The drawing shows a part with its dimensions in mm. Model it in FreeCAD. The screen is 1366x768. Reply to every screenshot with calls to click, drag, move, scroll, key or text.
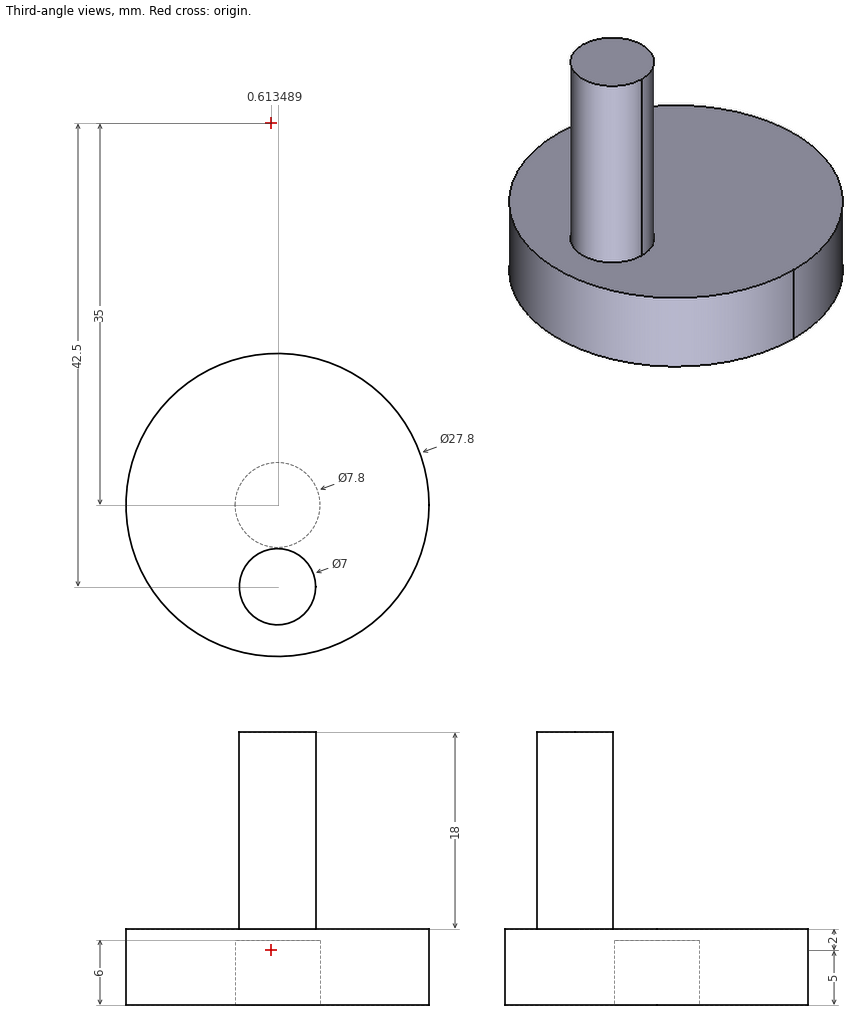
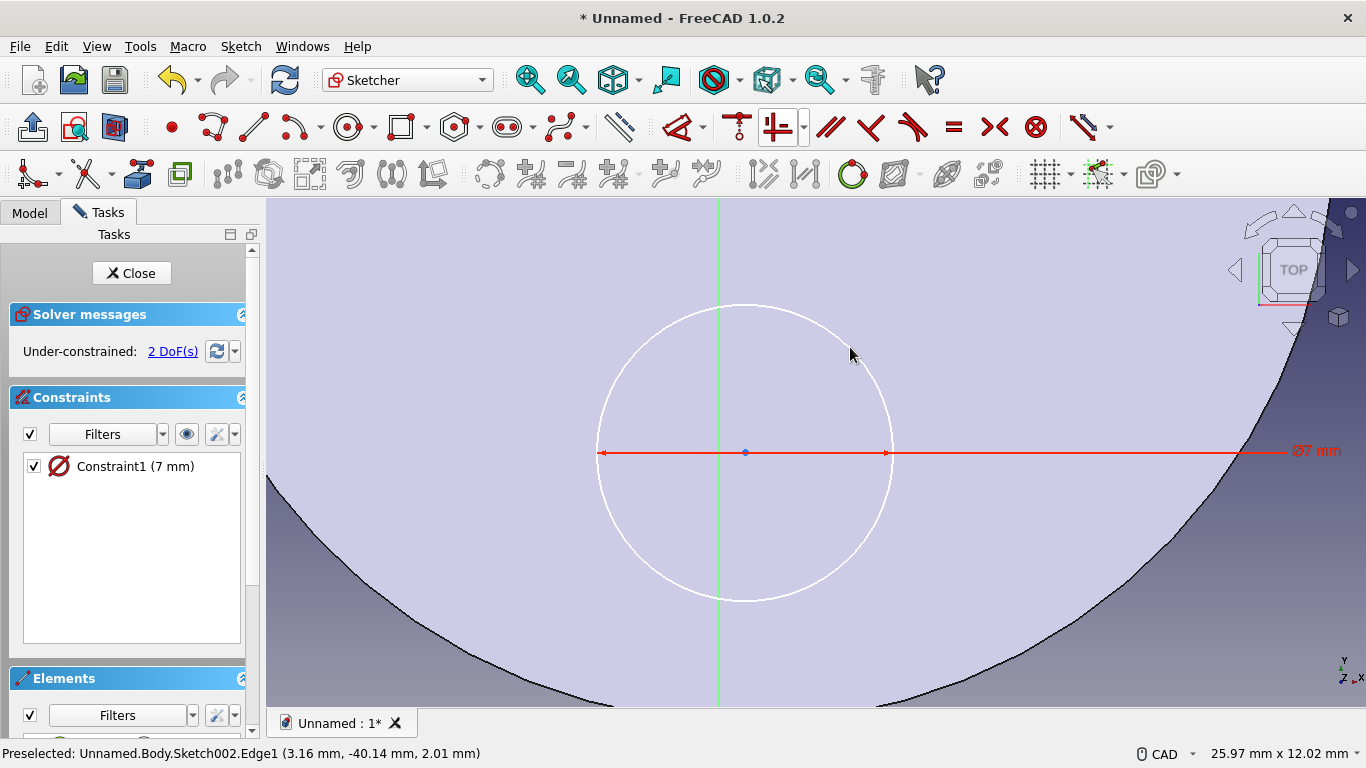
click(676, 128)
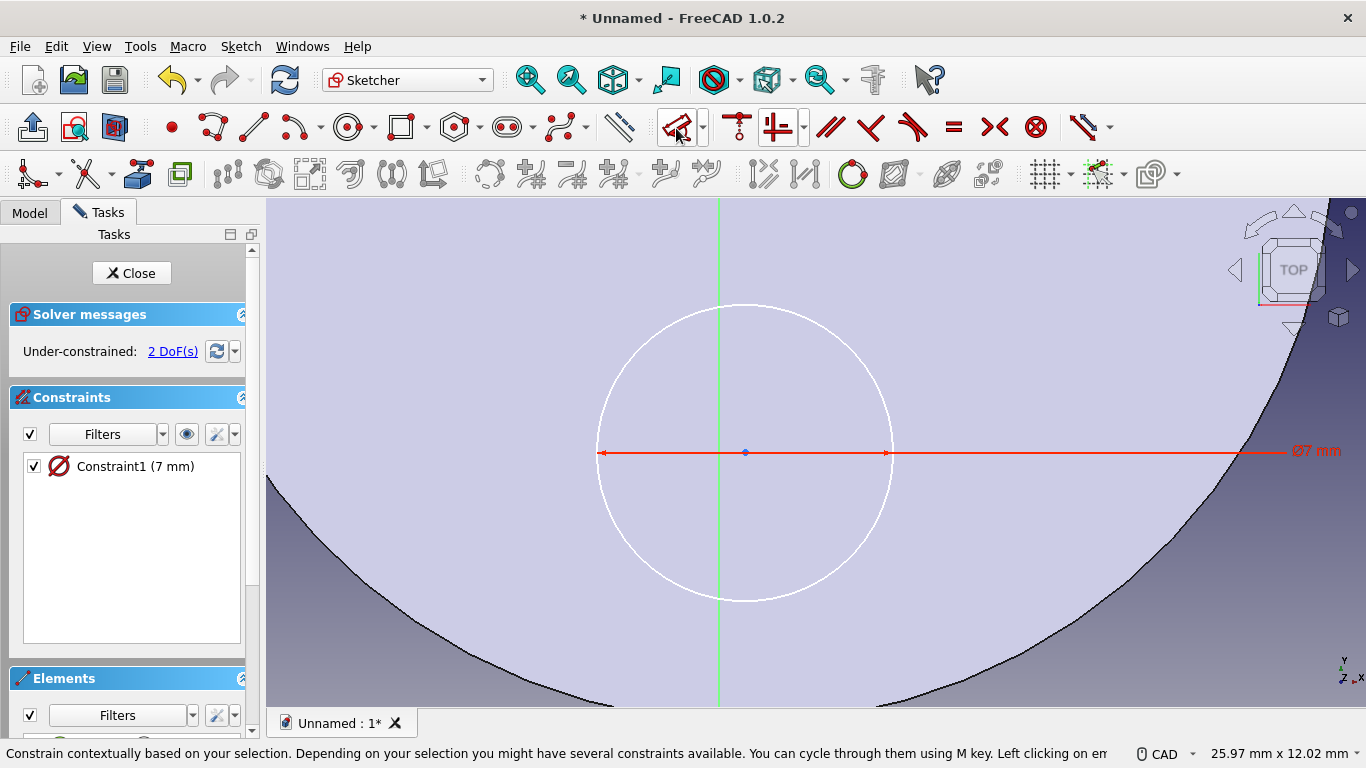
click(745, 453)
click(685, 339)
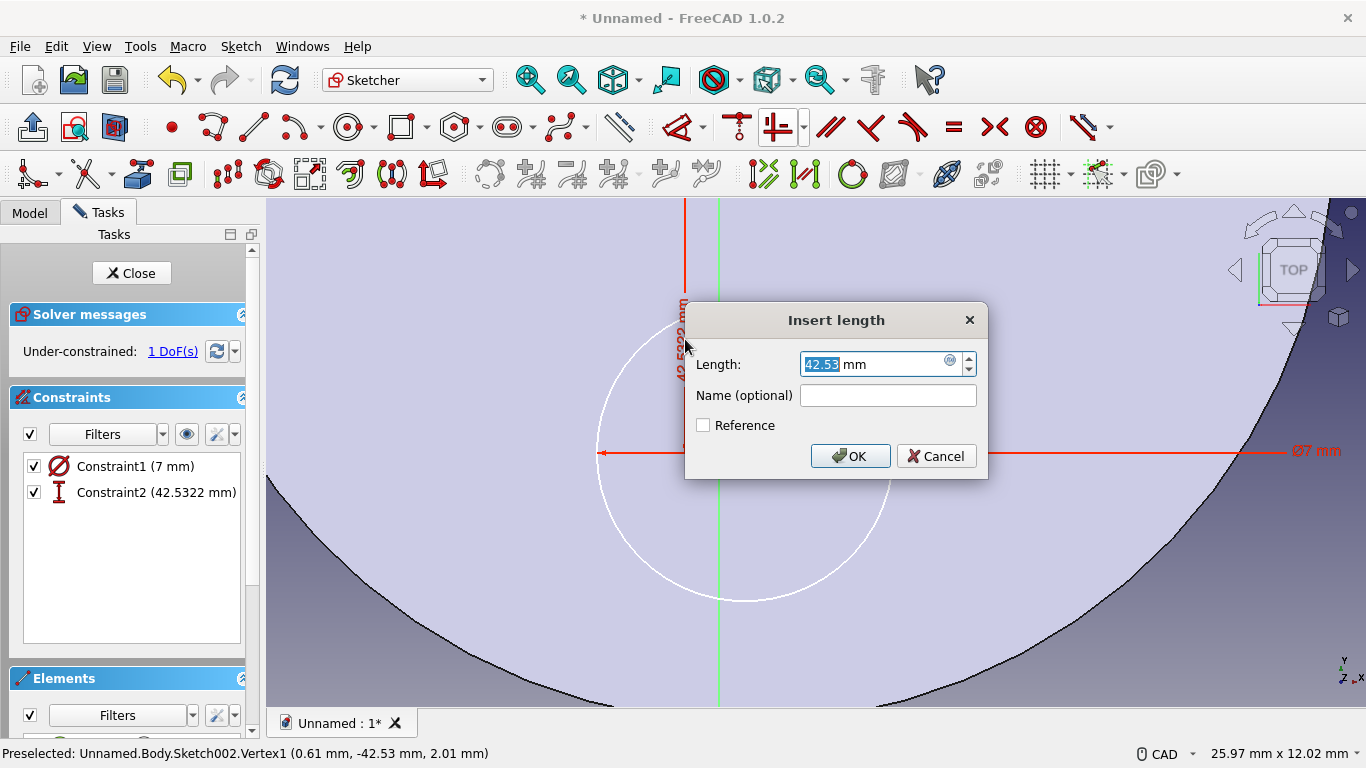
text(42.5)
key(Return)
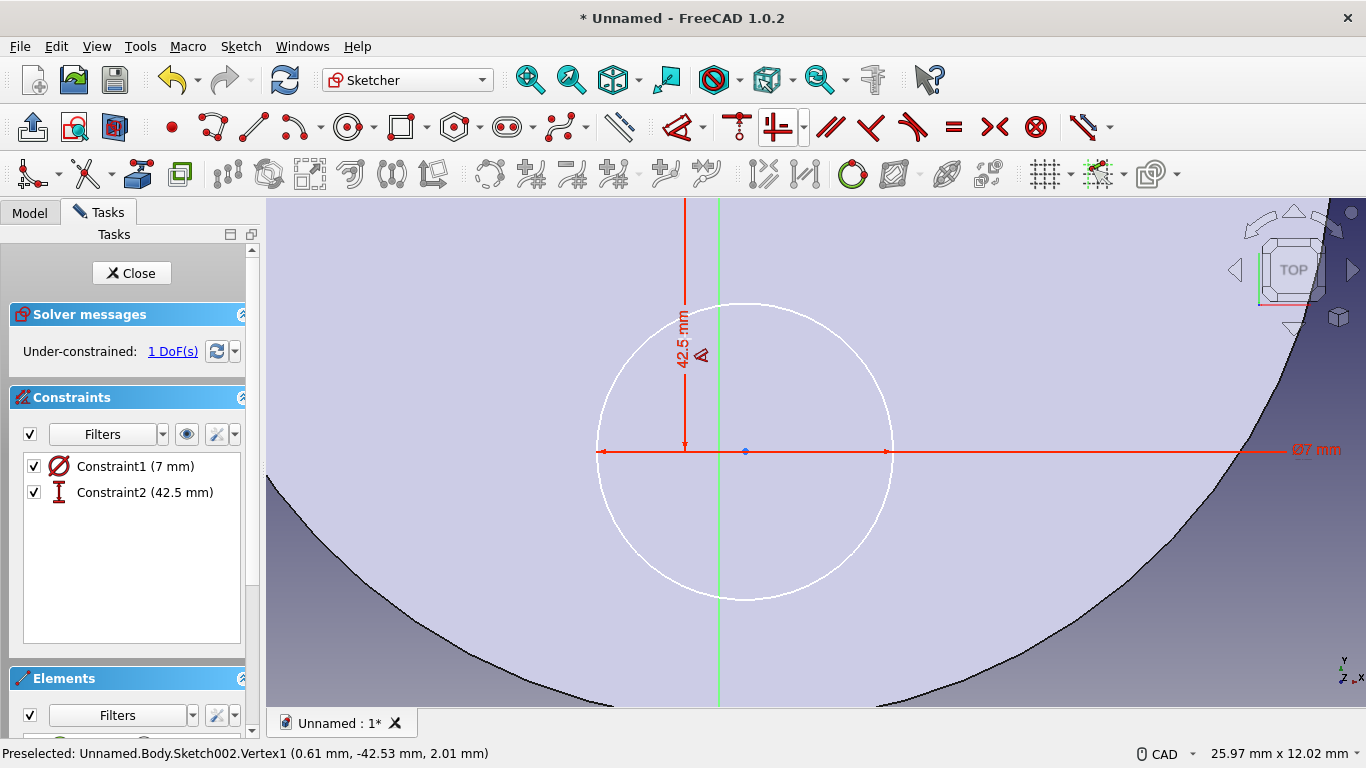
scroll(745, 452, up, 3)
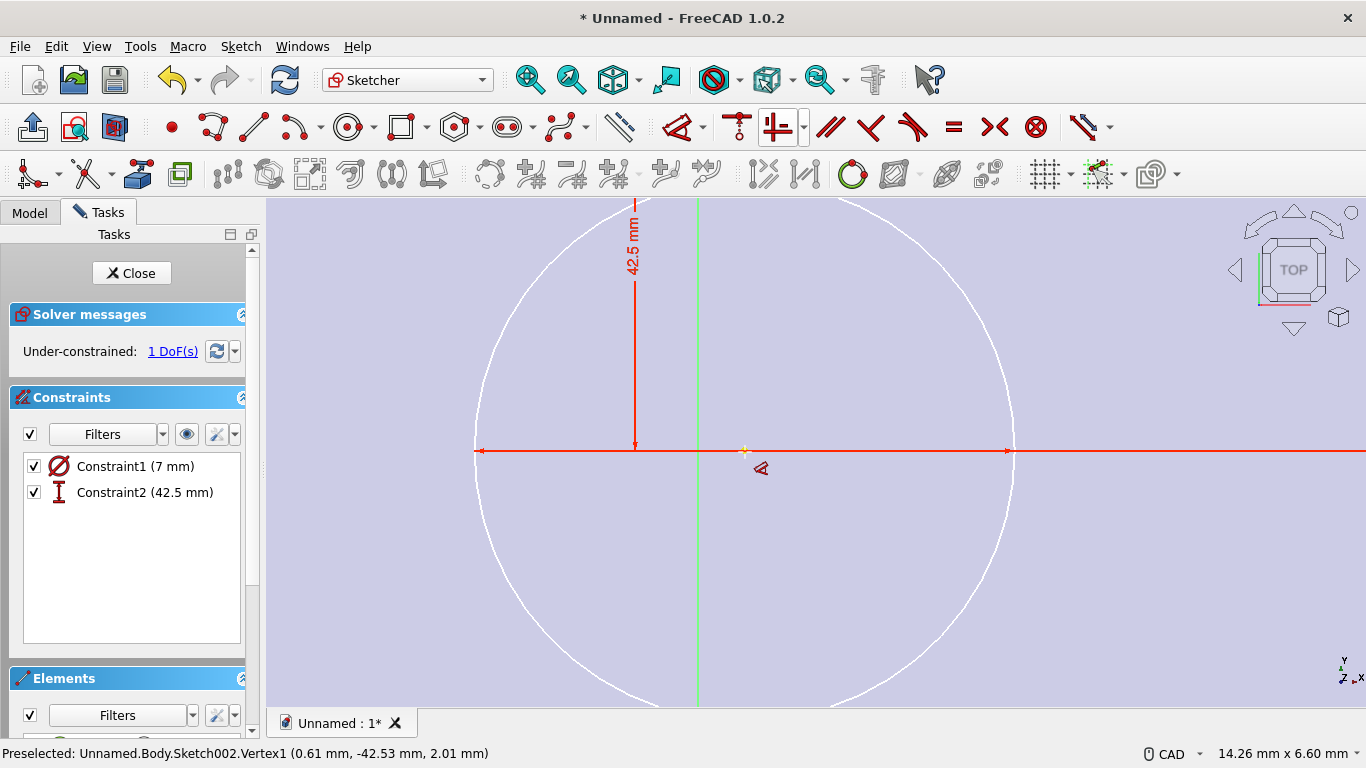
click(745, 451)
click(721, 485)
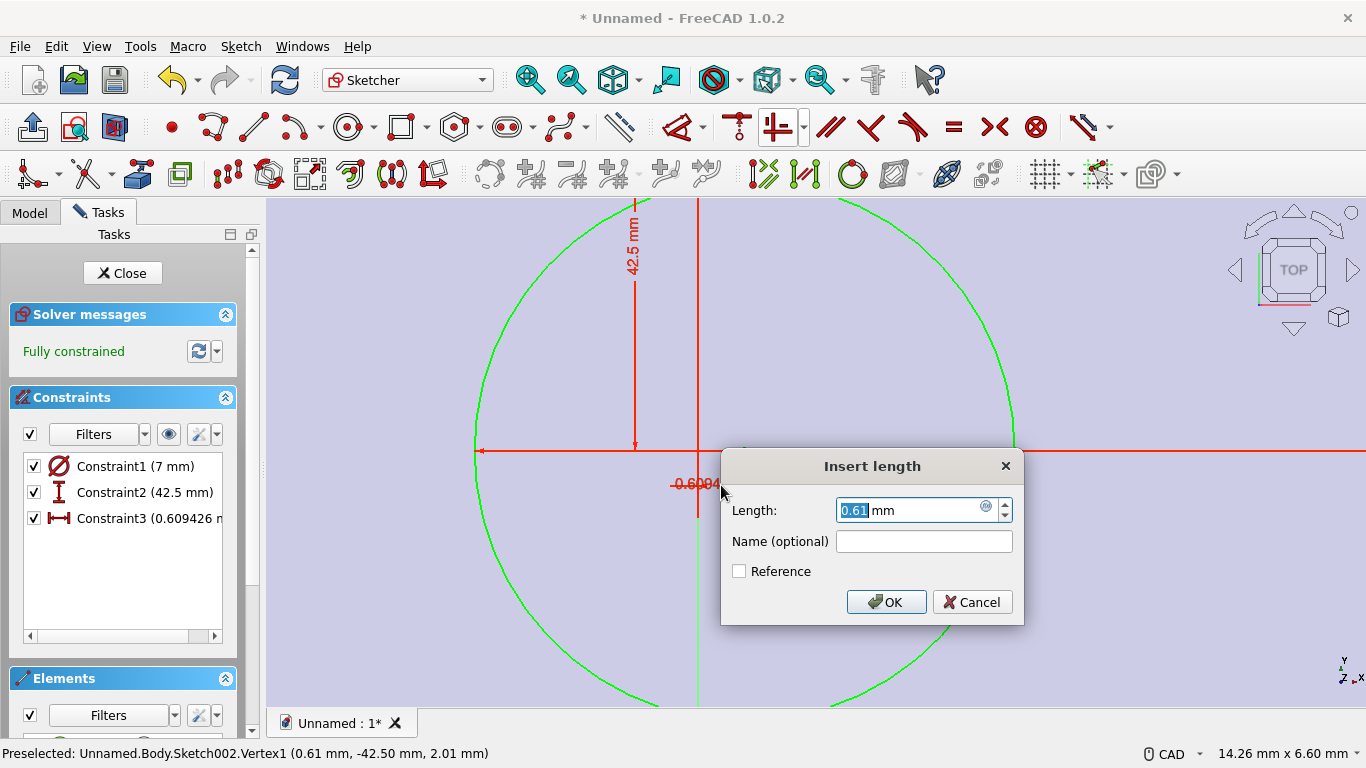
text(0.613489)
key(Return)
key(Escape)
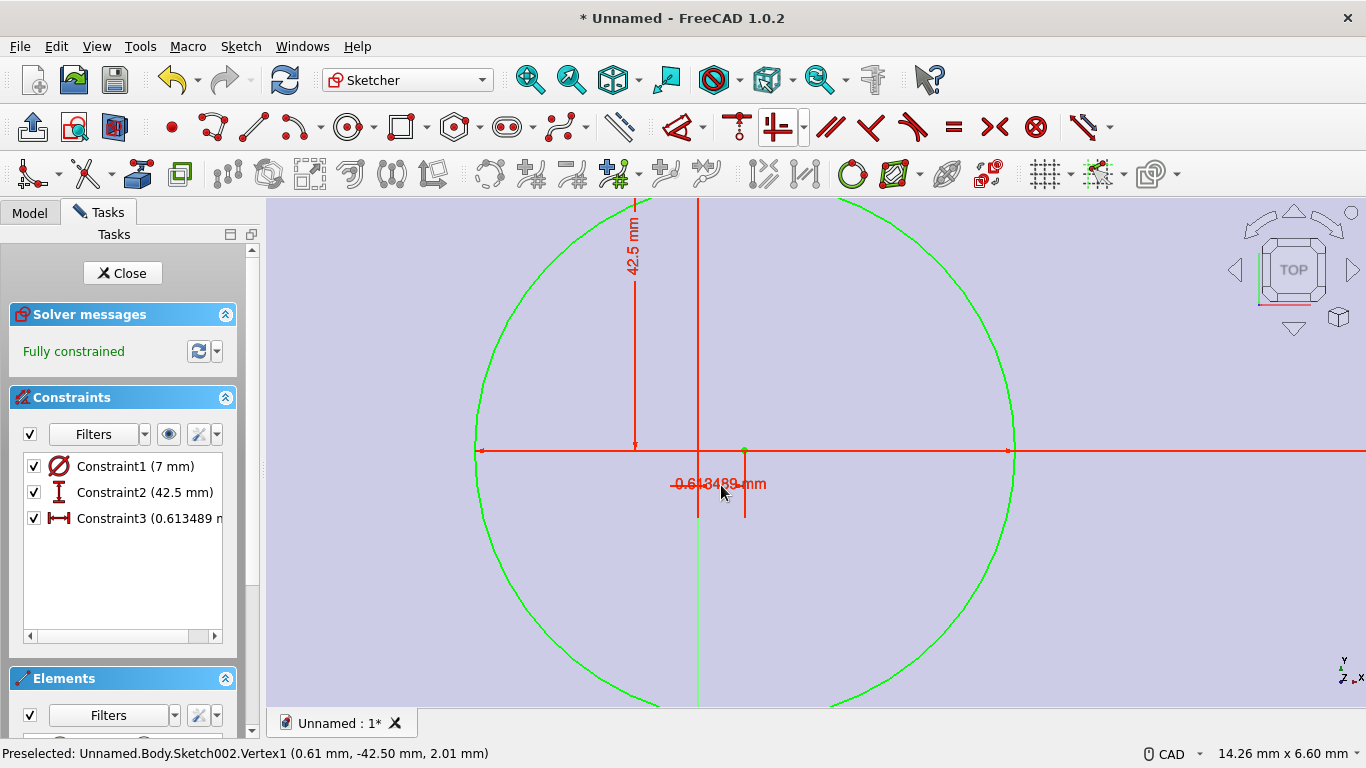
click(123, 273)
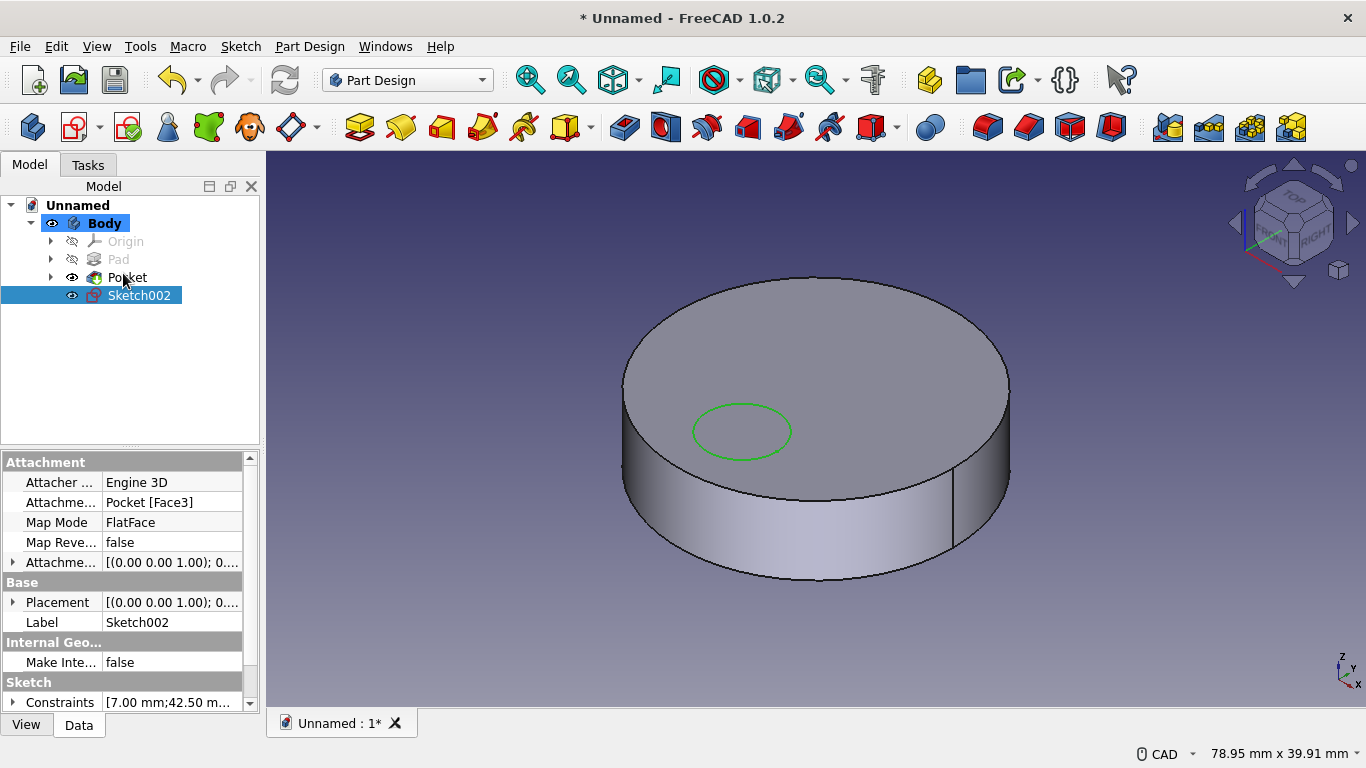
click(360, 128)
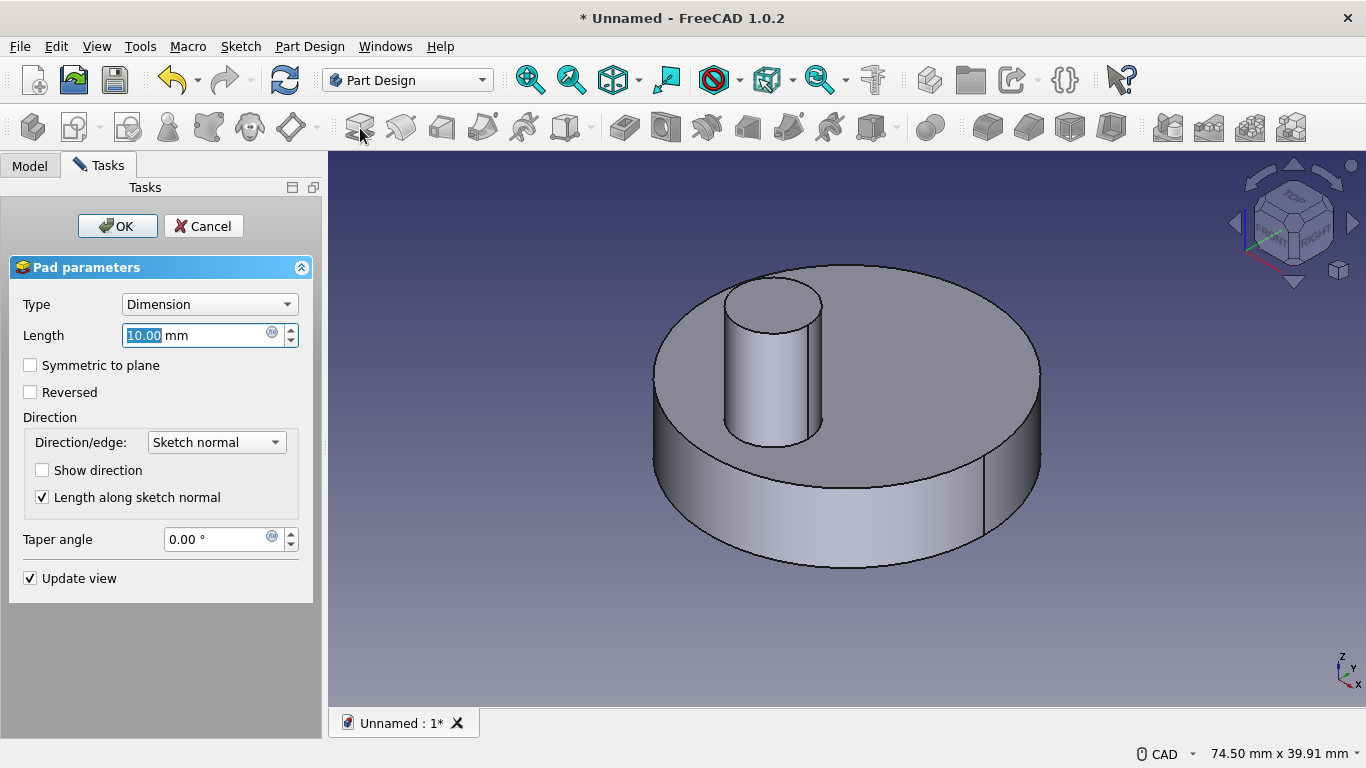
text(18)
key(Tab)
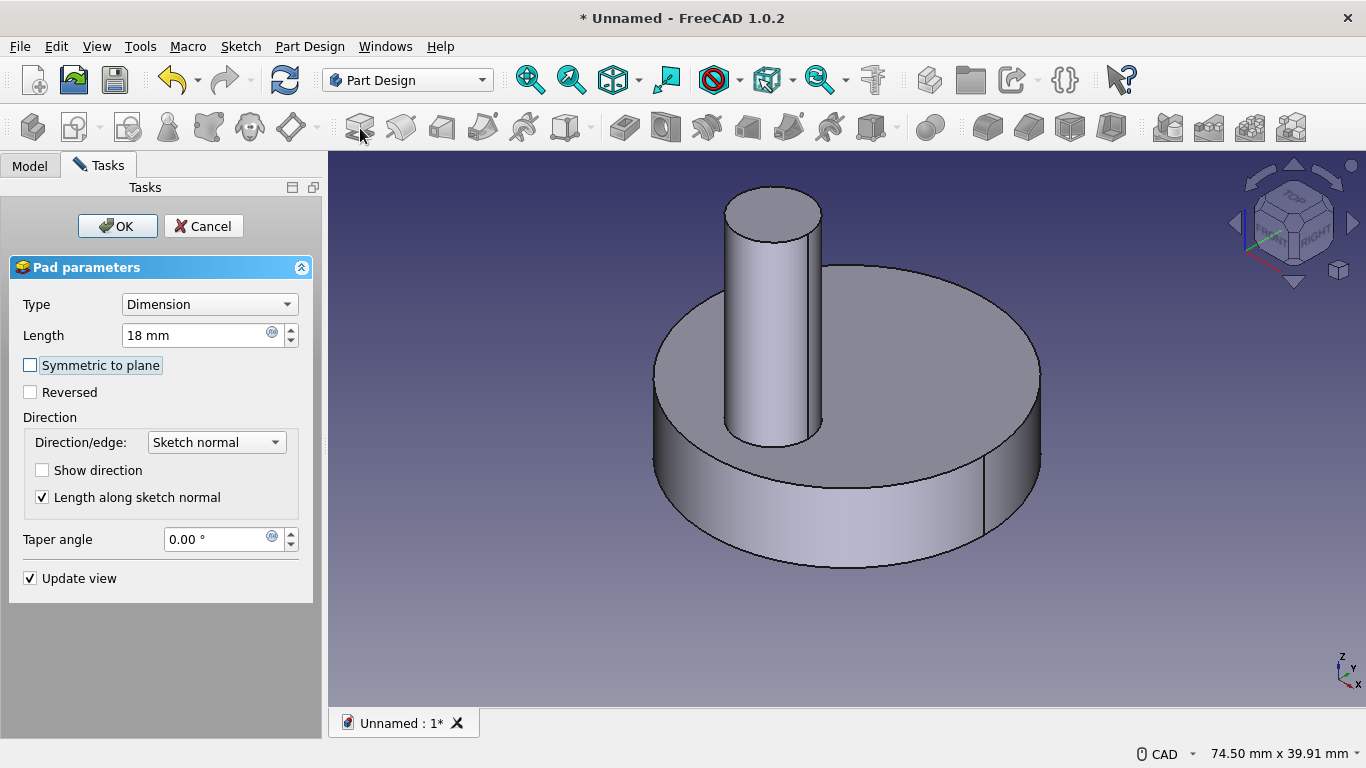
click(118, 226)